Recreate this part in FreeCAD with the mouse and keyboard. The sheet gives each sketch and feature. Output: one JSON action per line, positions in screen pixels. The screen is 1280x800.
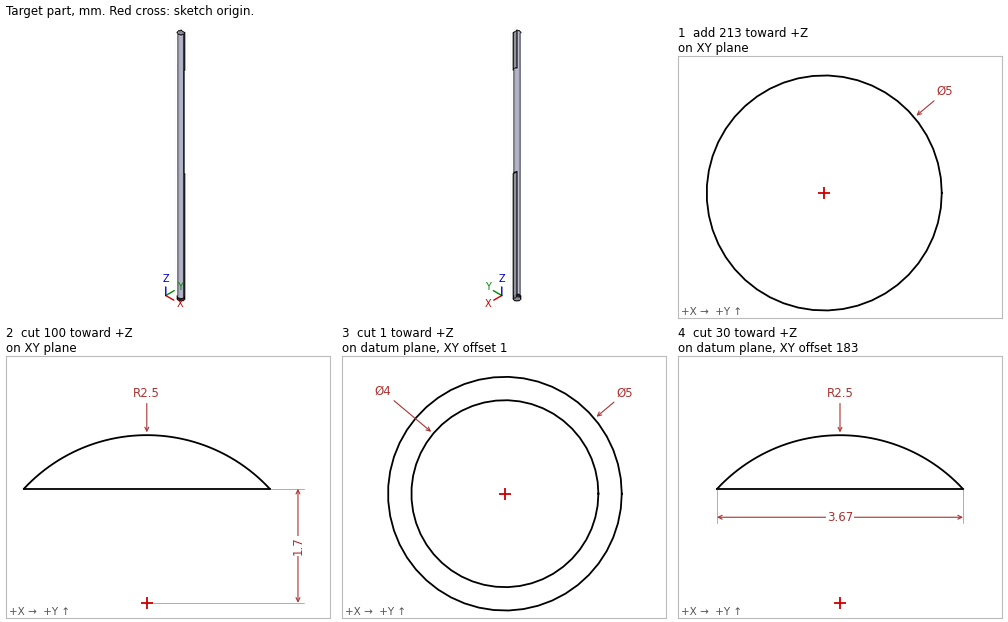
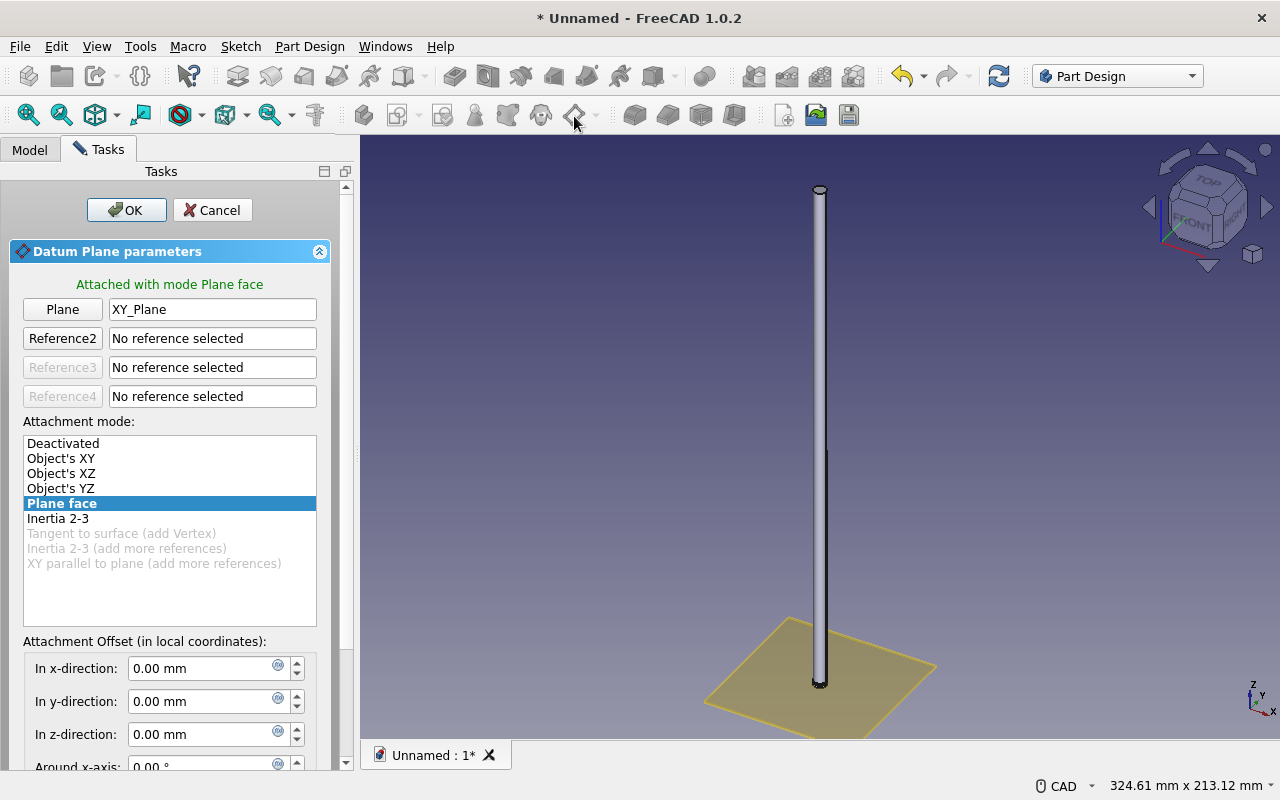
{"action": "triple_click", "coordinate": [210, 734]}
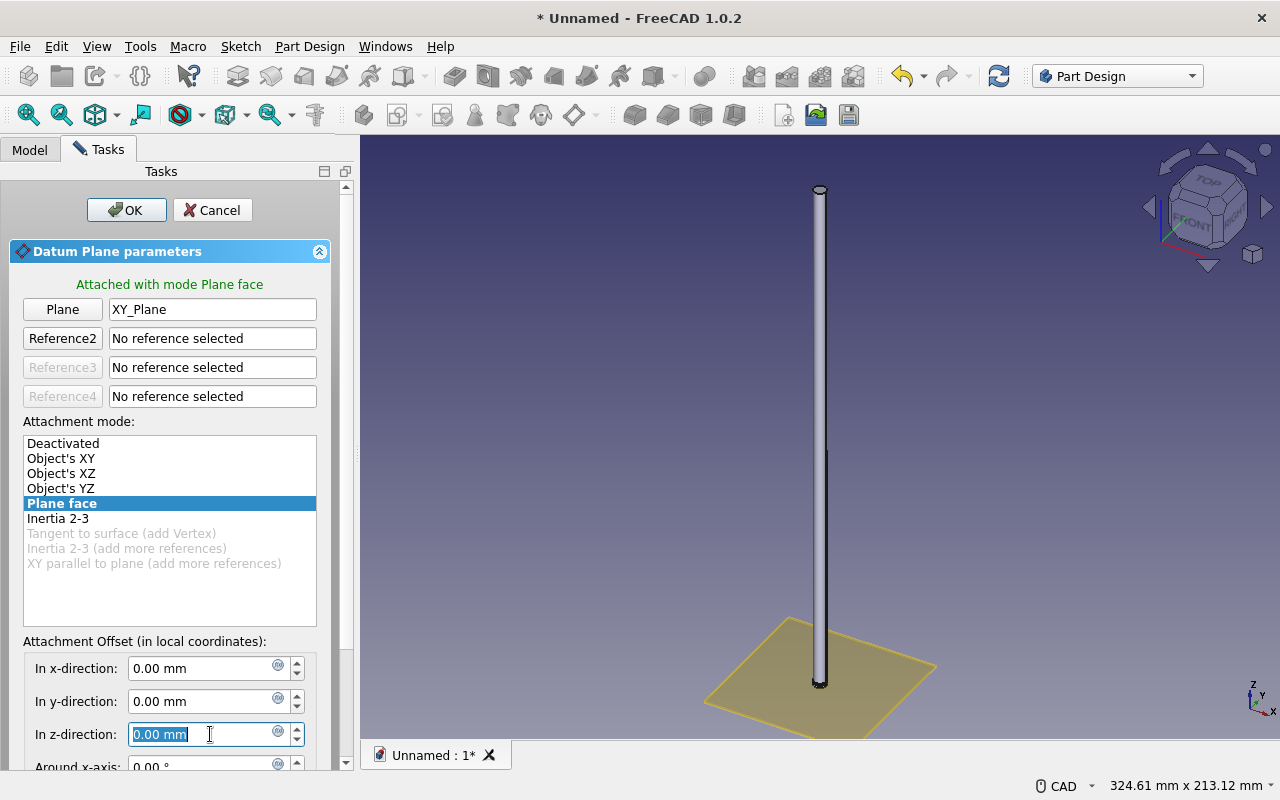
{"action": "type", "text": "183"}
{"action": "key", "text": "Tab"}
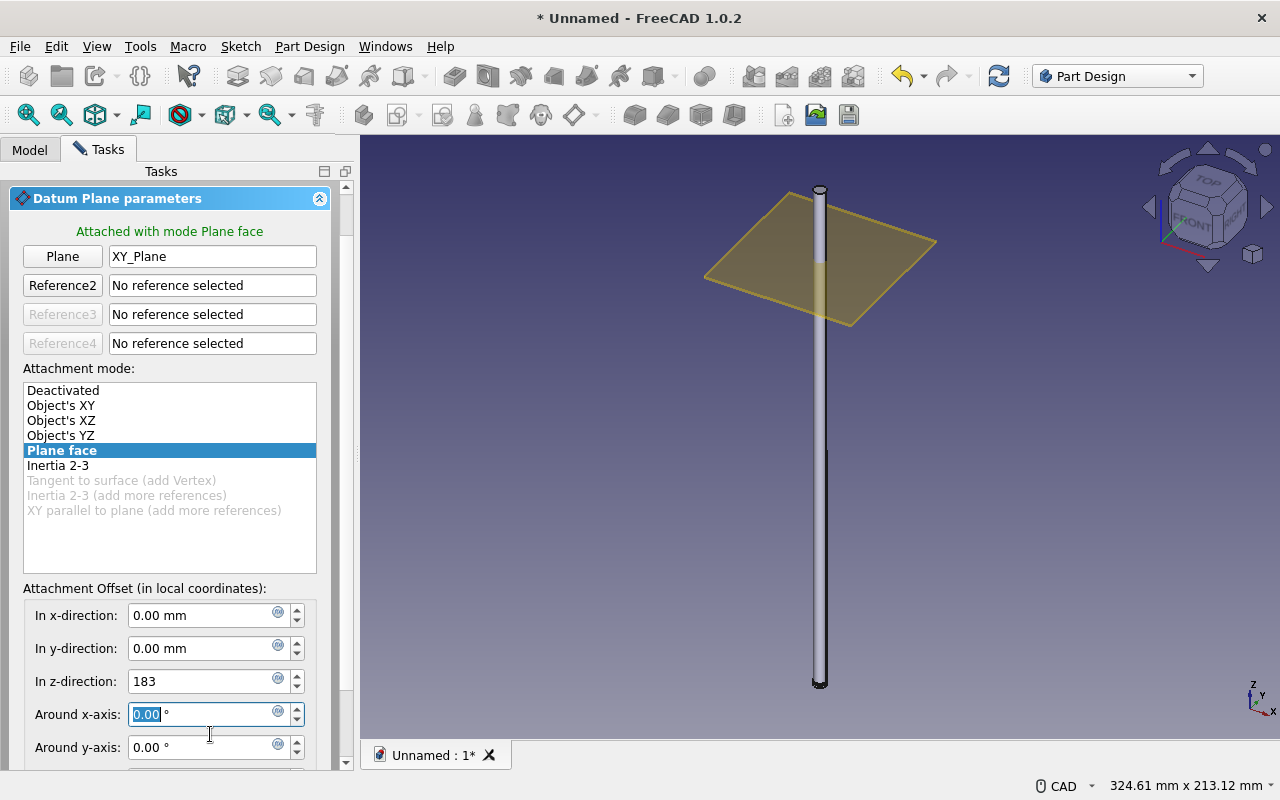
{"action": "scroll", "coordinate": [346, 476], "scroll_direction": "up", "scroll_amount": 2}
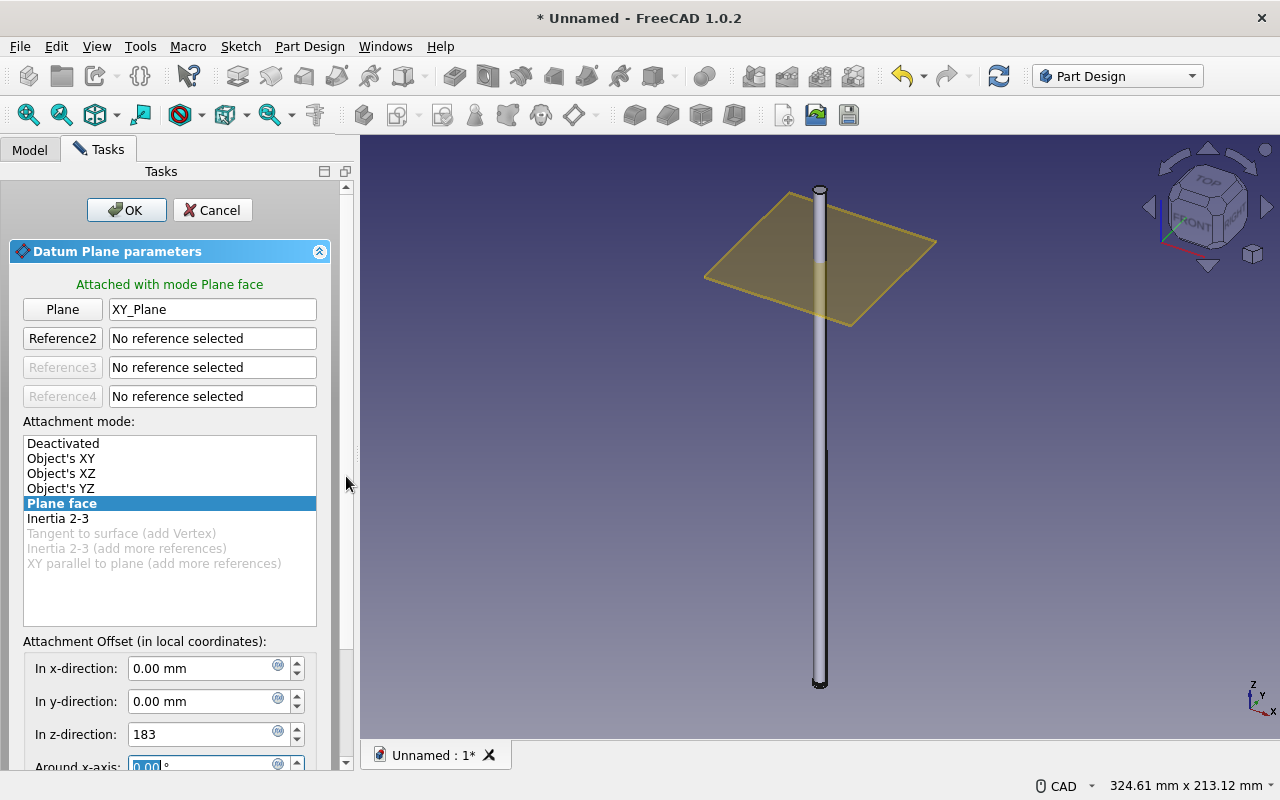
{"action": "left_click", "coordinate": [127, 210]}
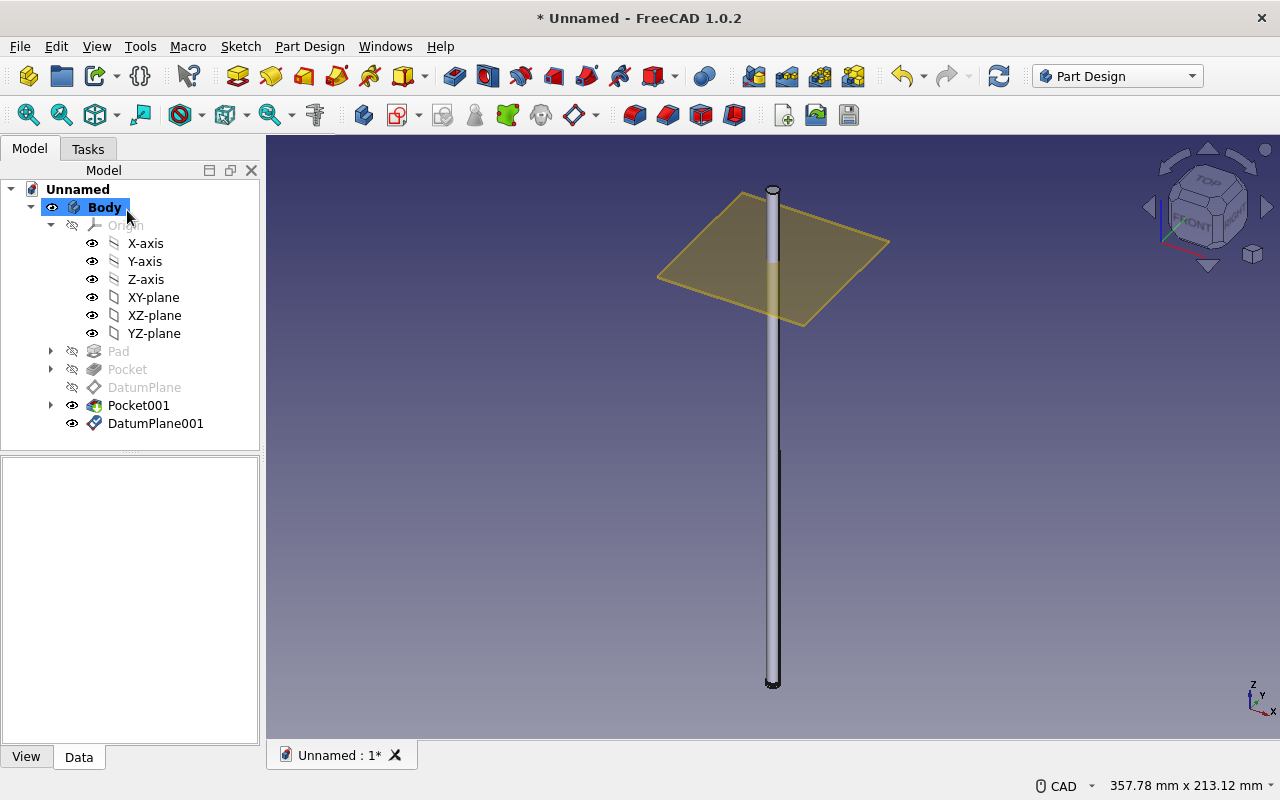
{"action": "left_click", "coordinate": [117, 423]}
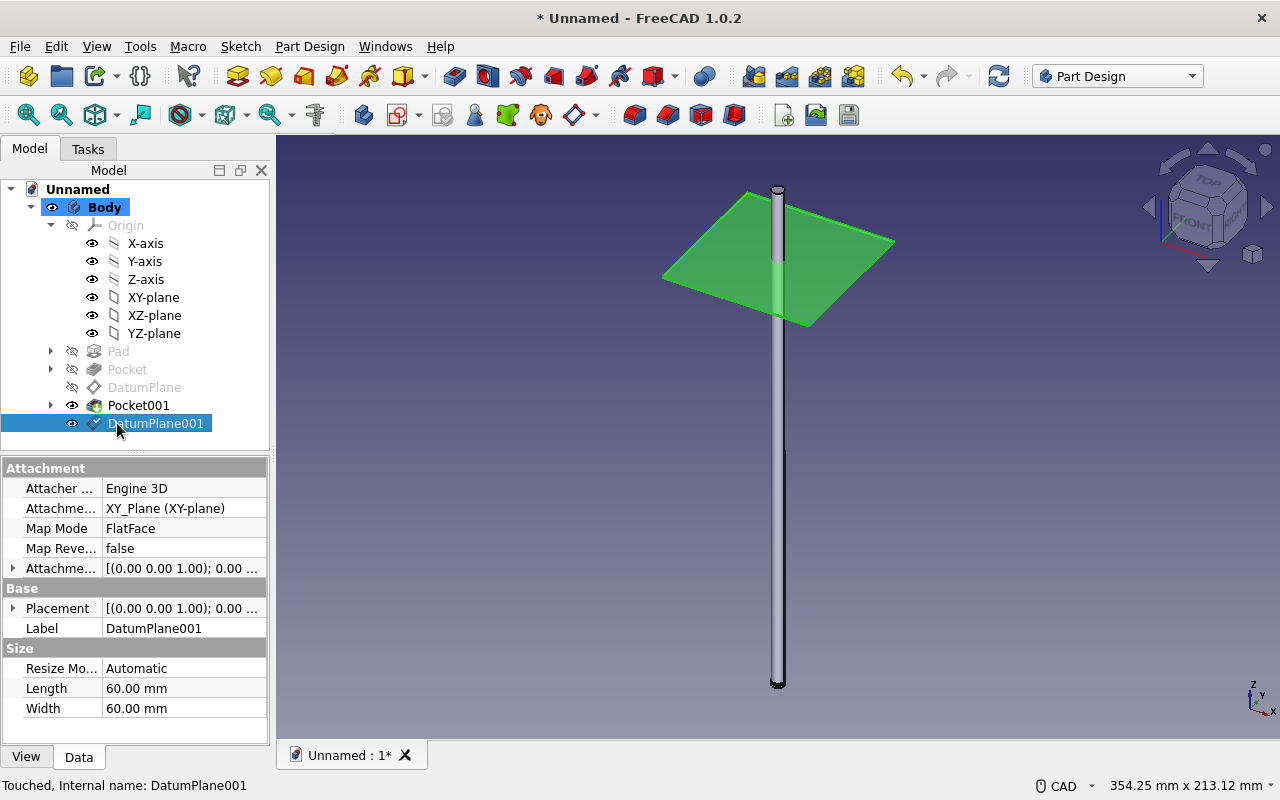
{"action": "left_click", "coordinate": [396, 116]}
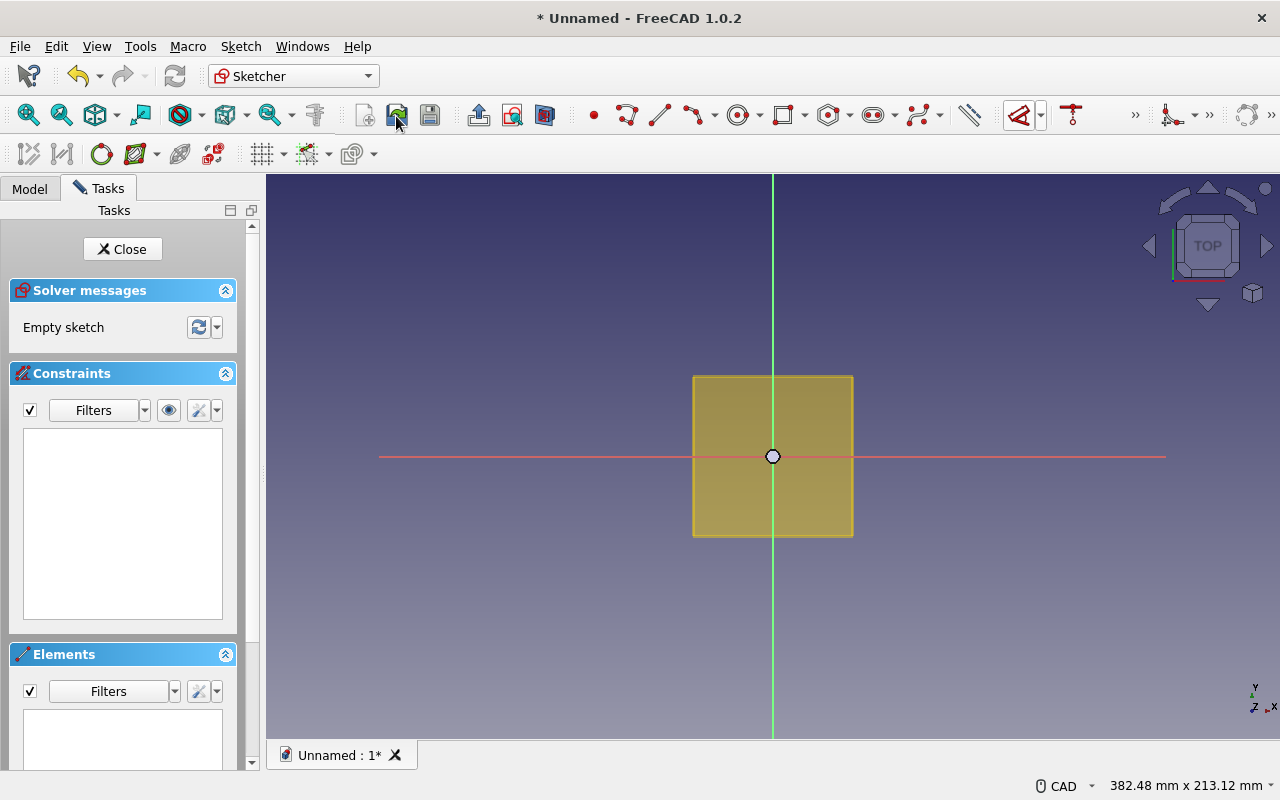
{"action": "left_click", "coordinate": [545, 116]}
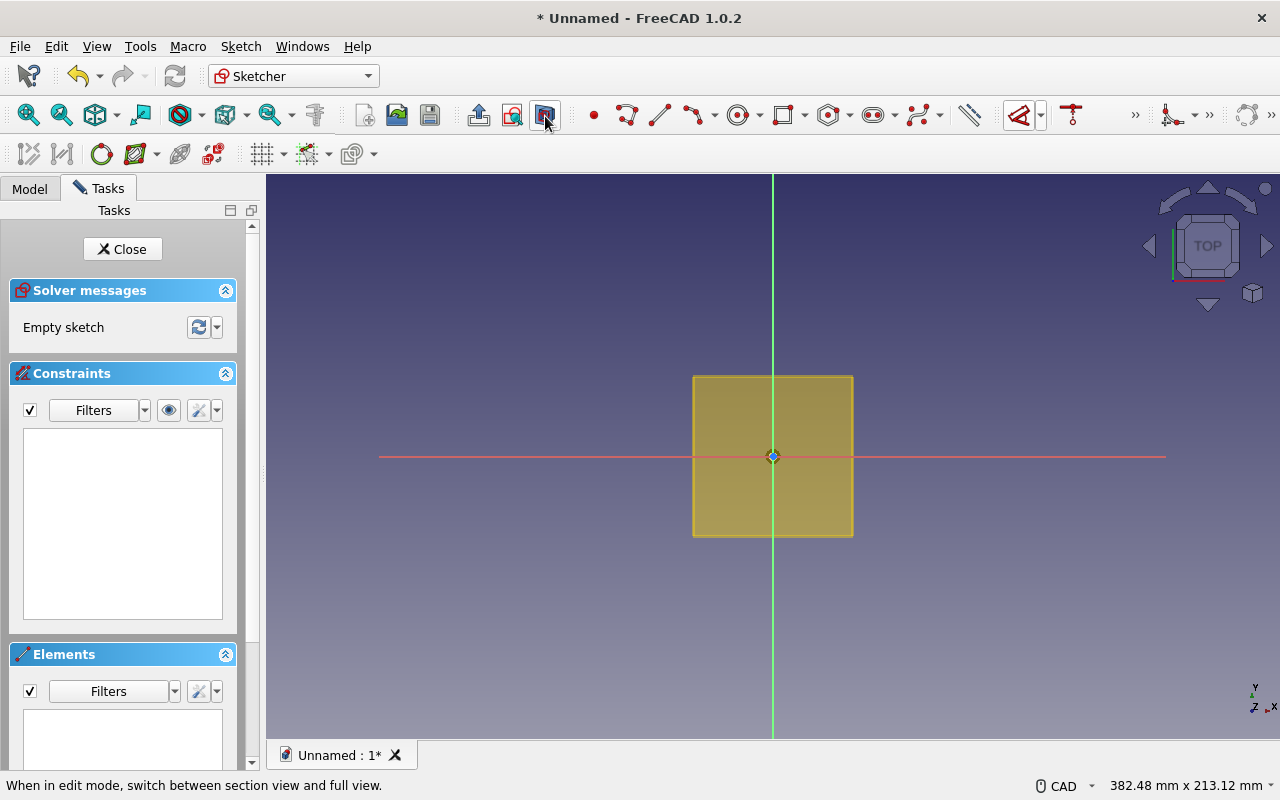
{"action": "scroll", "coordinate": [777, 453], "scroll_direction": "up", "scroll_amount": 15}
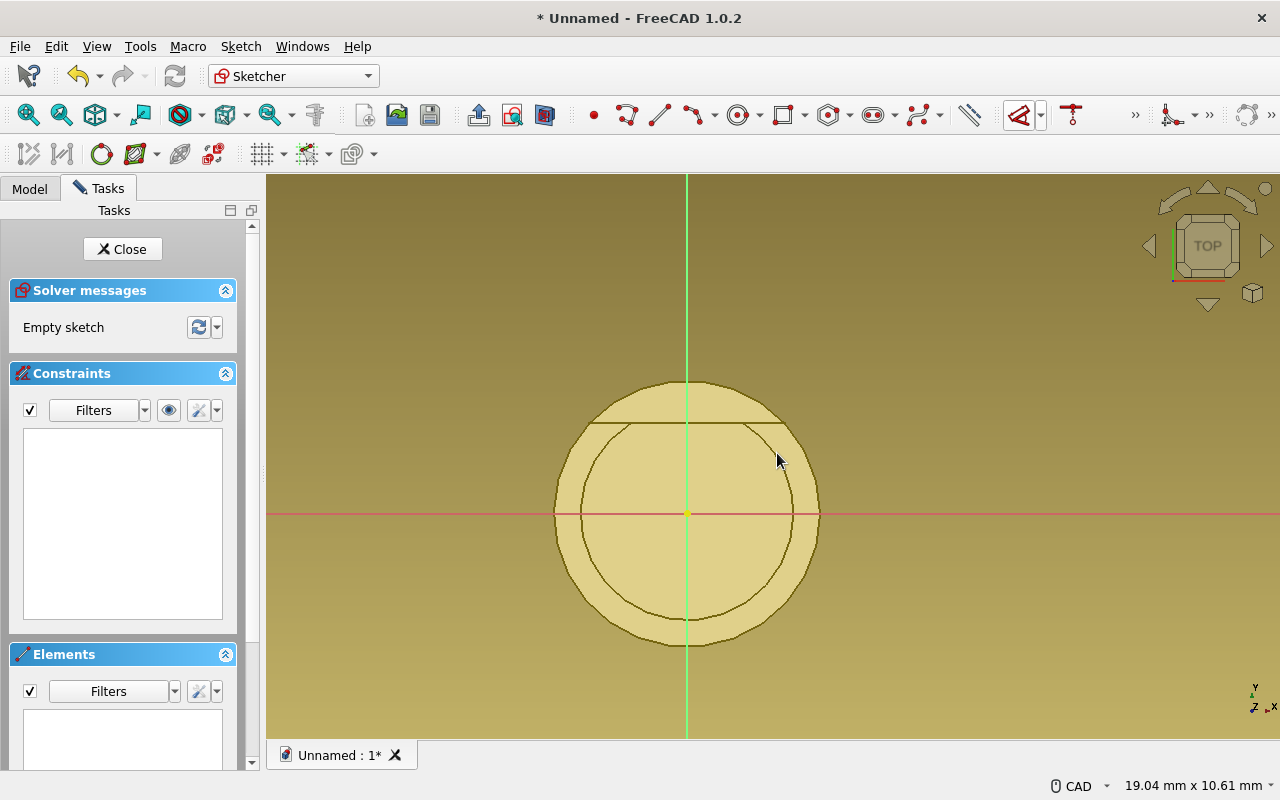
{"action": "scroll", "coordinate": [677, 442], "scroll_direction": "up", "scroll_amount": 5}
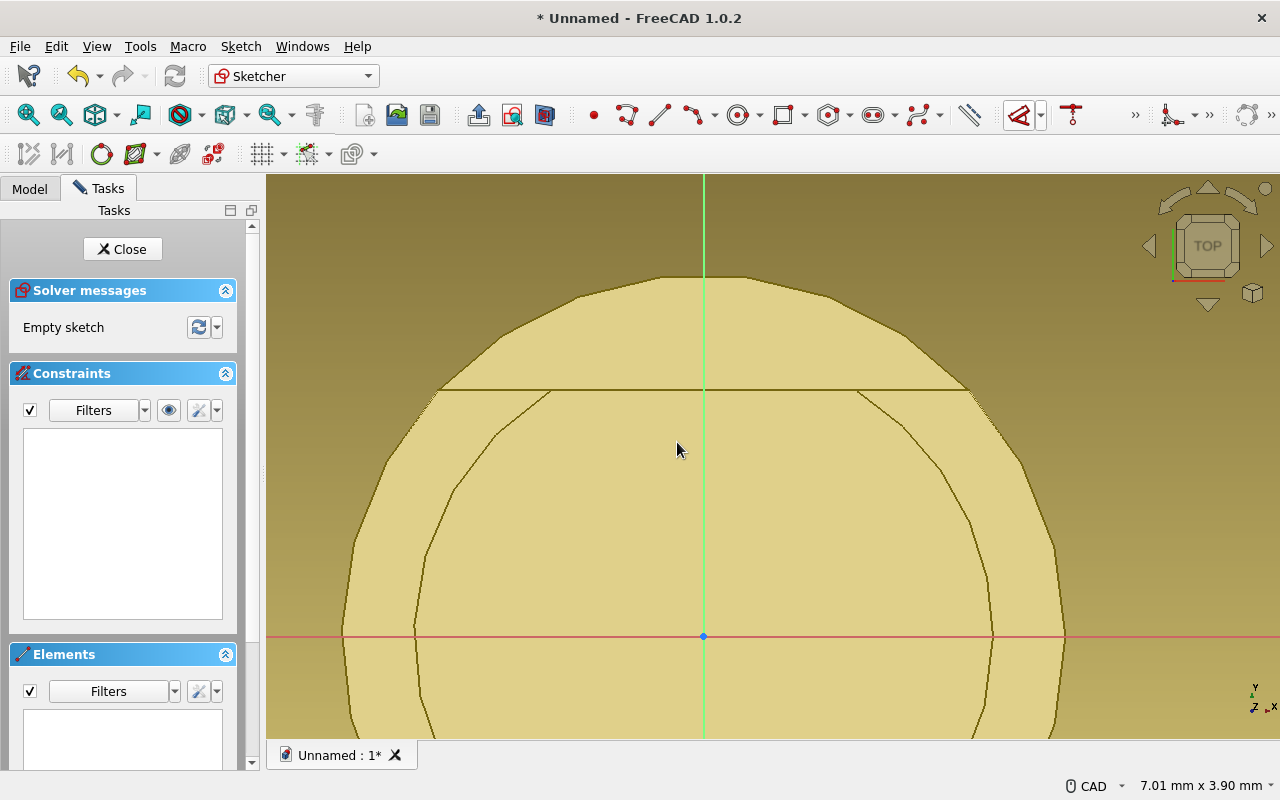
{"action": "key", "text": "g l"}